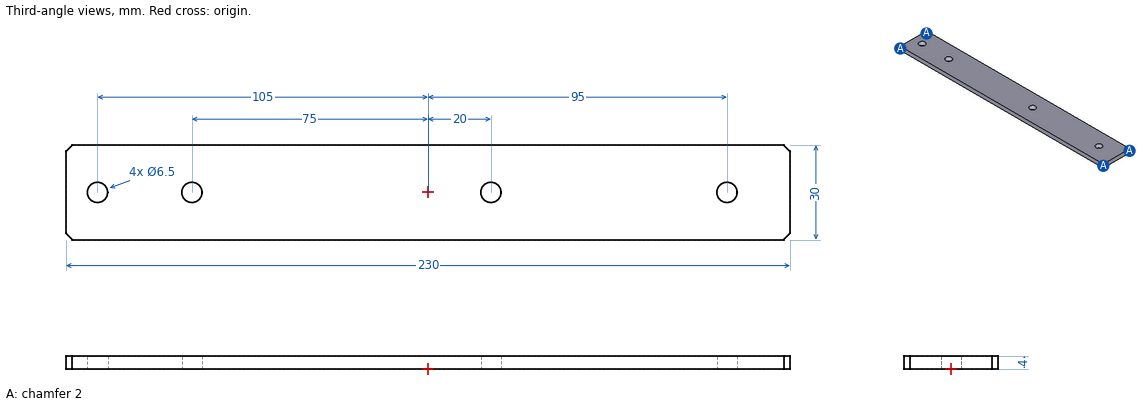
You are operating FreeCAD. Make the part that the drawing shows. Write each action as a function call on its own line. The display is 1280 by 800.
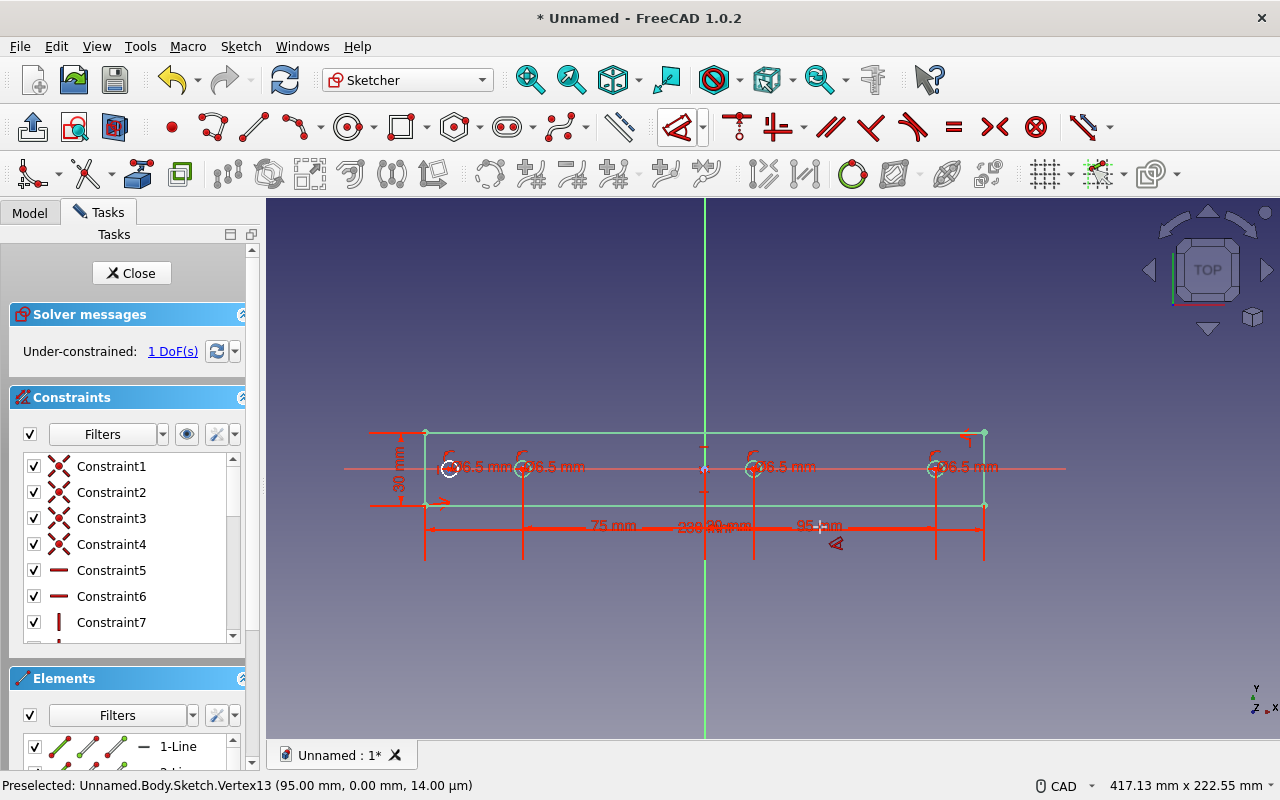
click(450, 469)
click(519, 527)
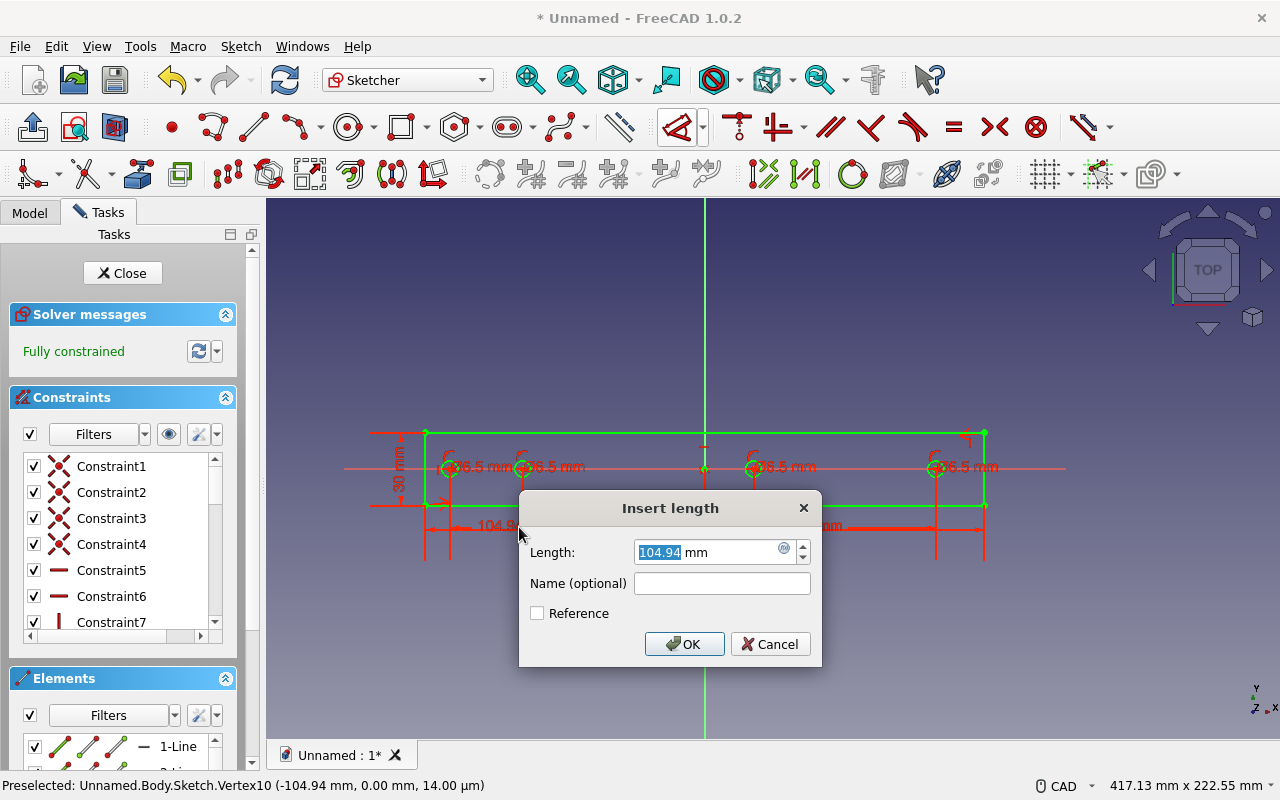
text(105)
key(Return)
key(Escape)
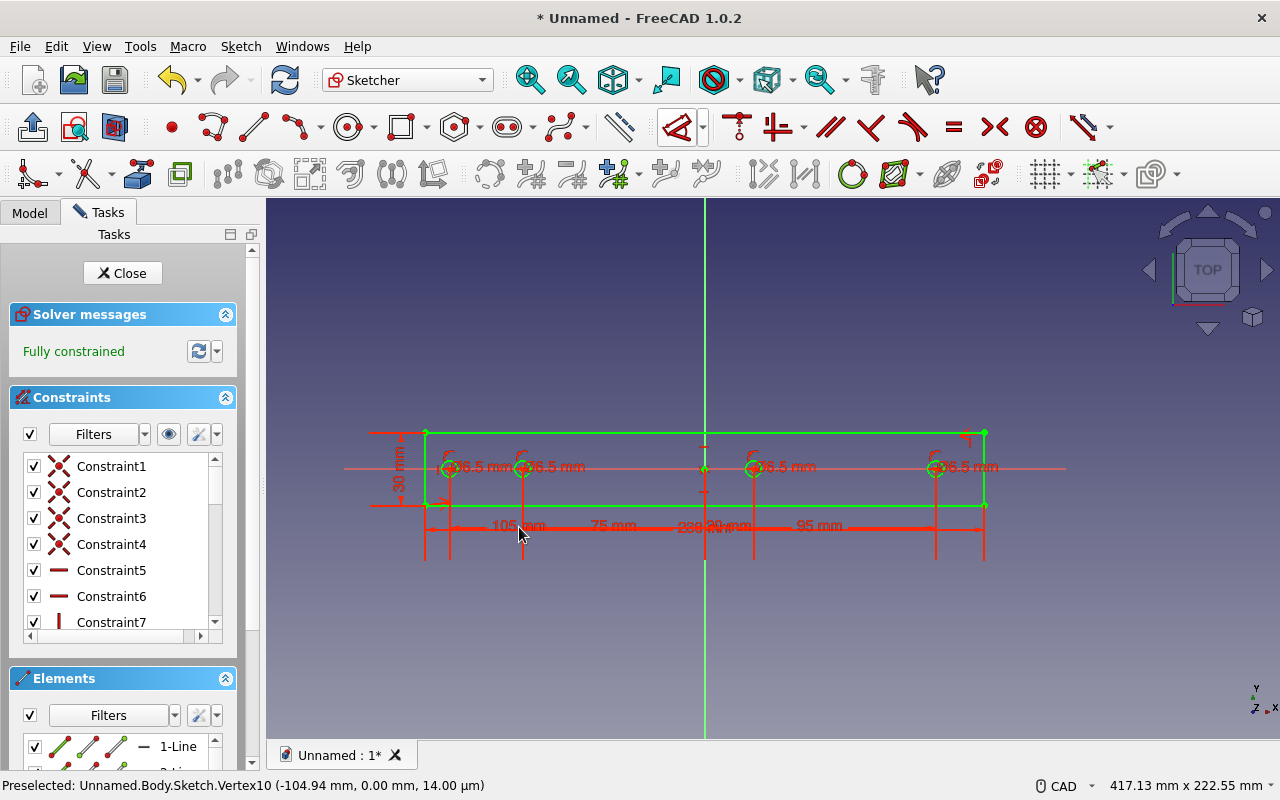
click(123, 273)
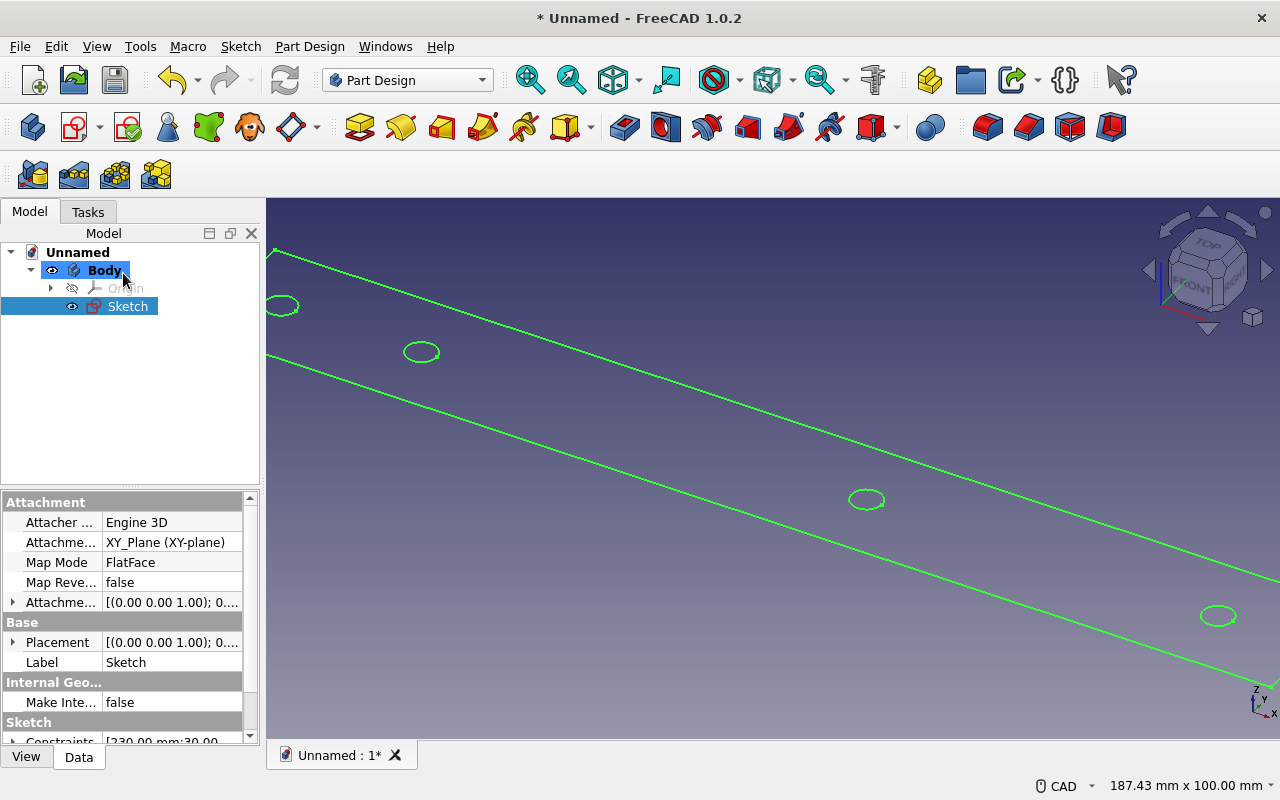
click(360, 128)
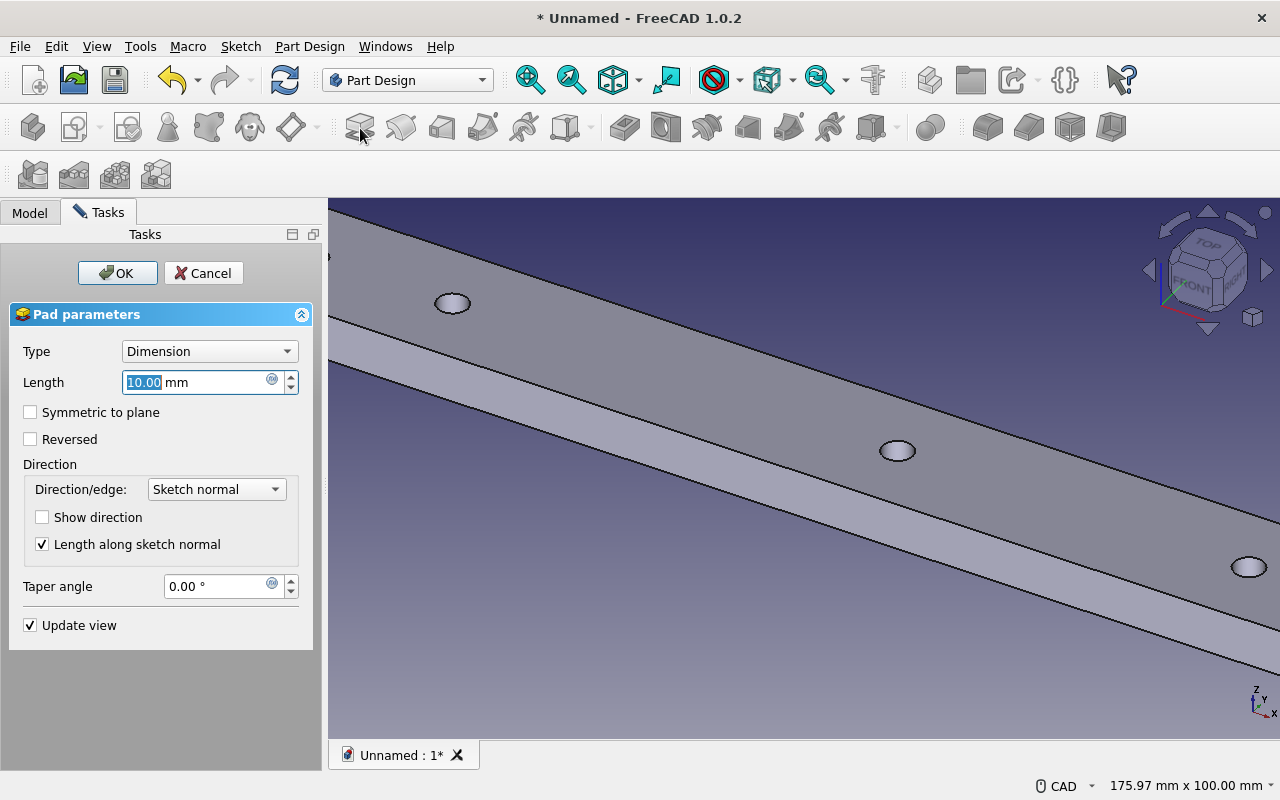
text(4)
key(Tab)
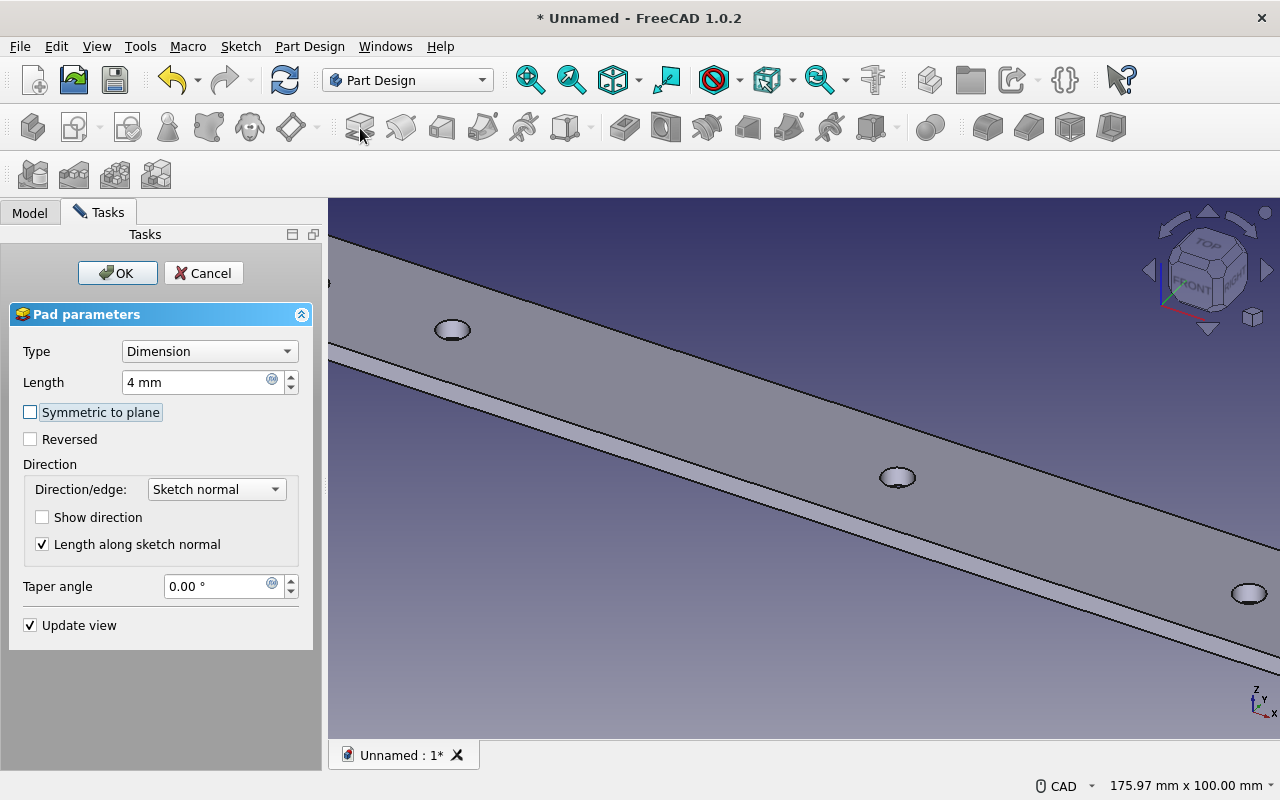
click(118, 273)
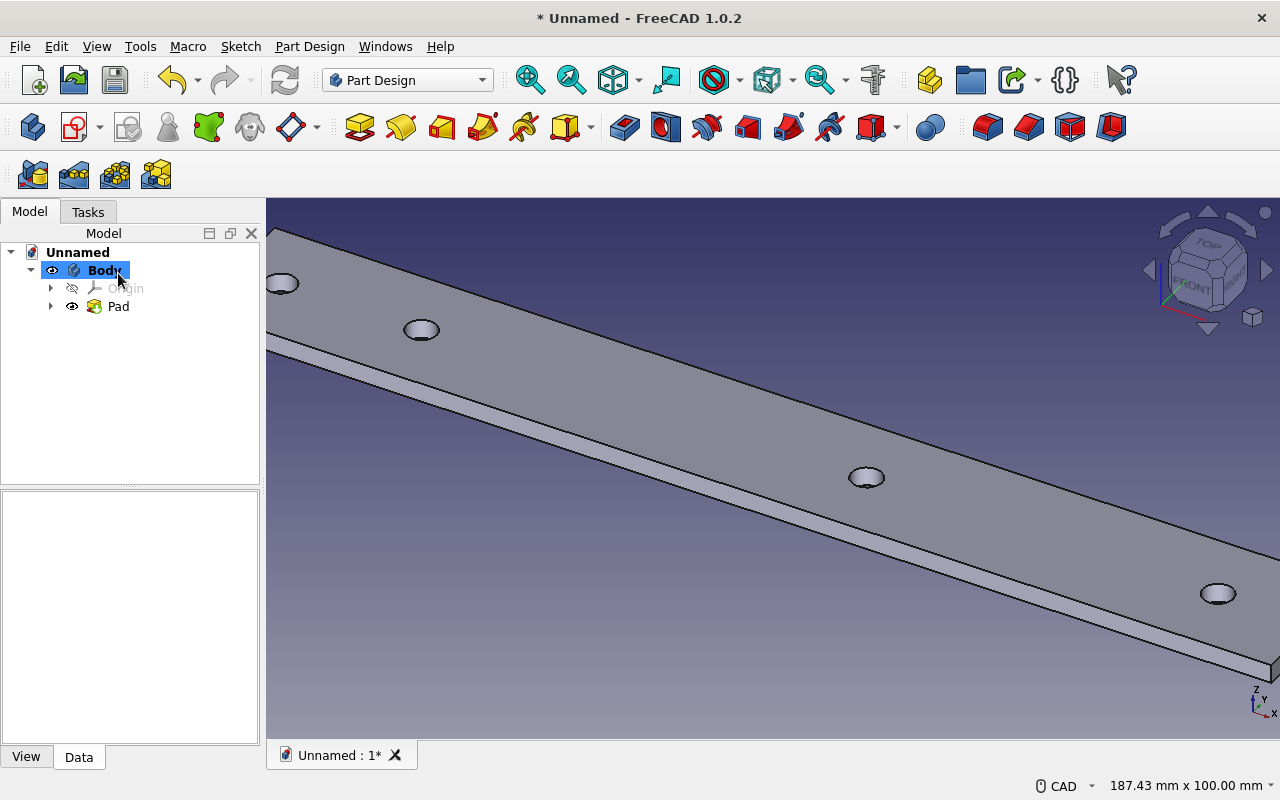
key(v)
key(f)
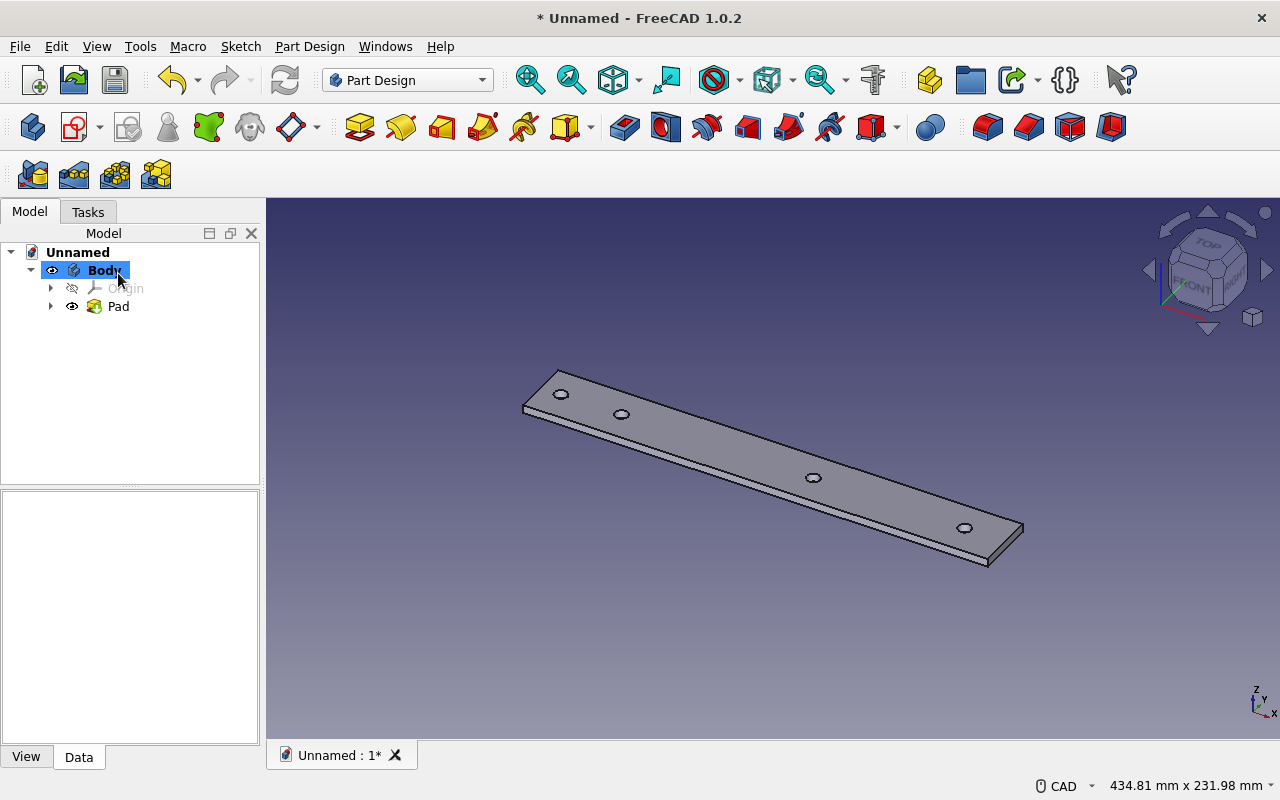
click(988, 564)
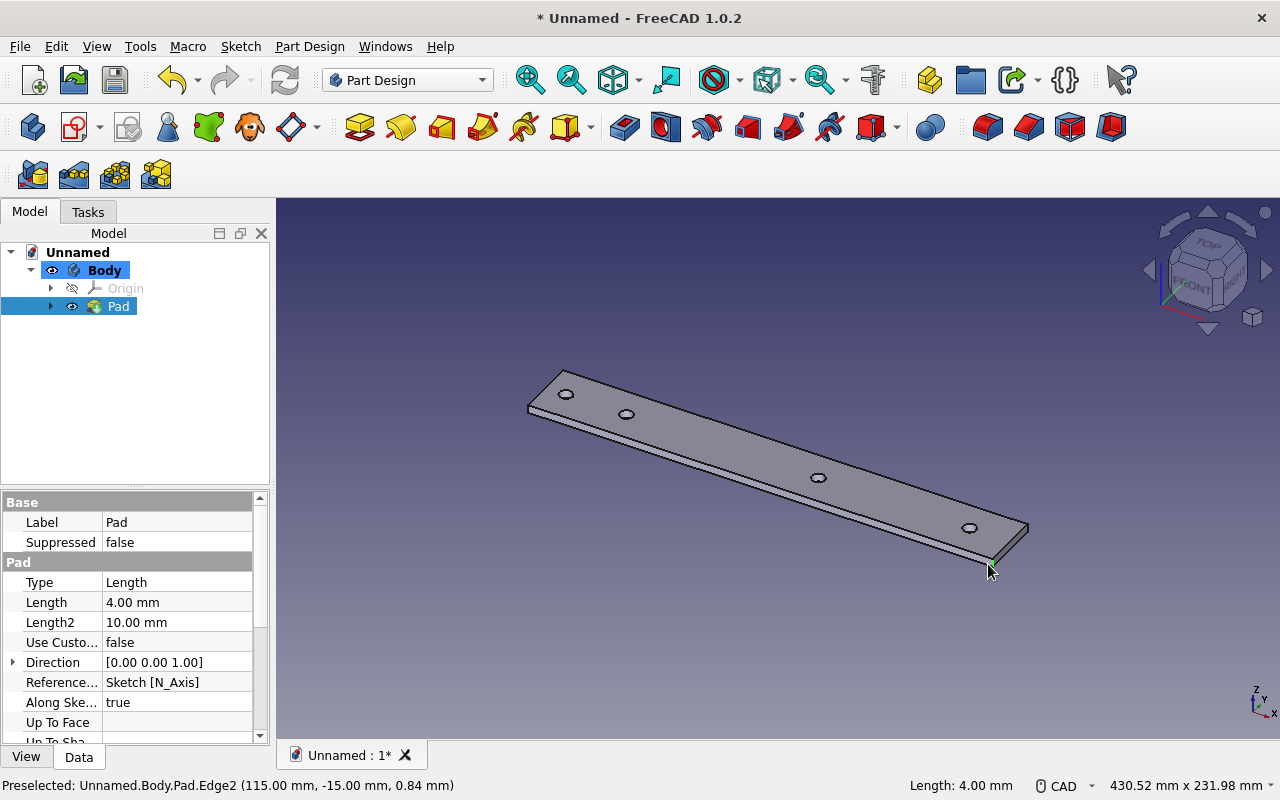
scroll(563, 373, up, 8)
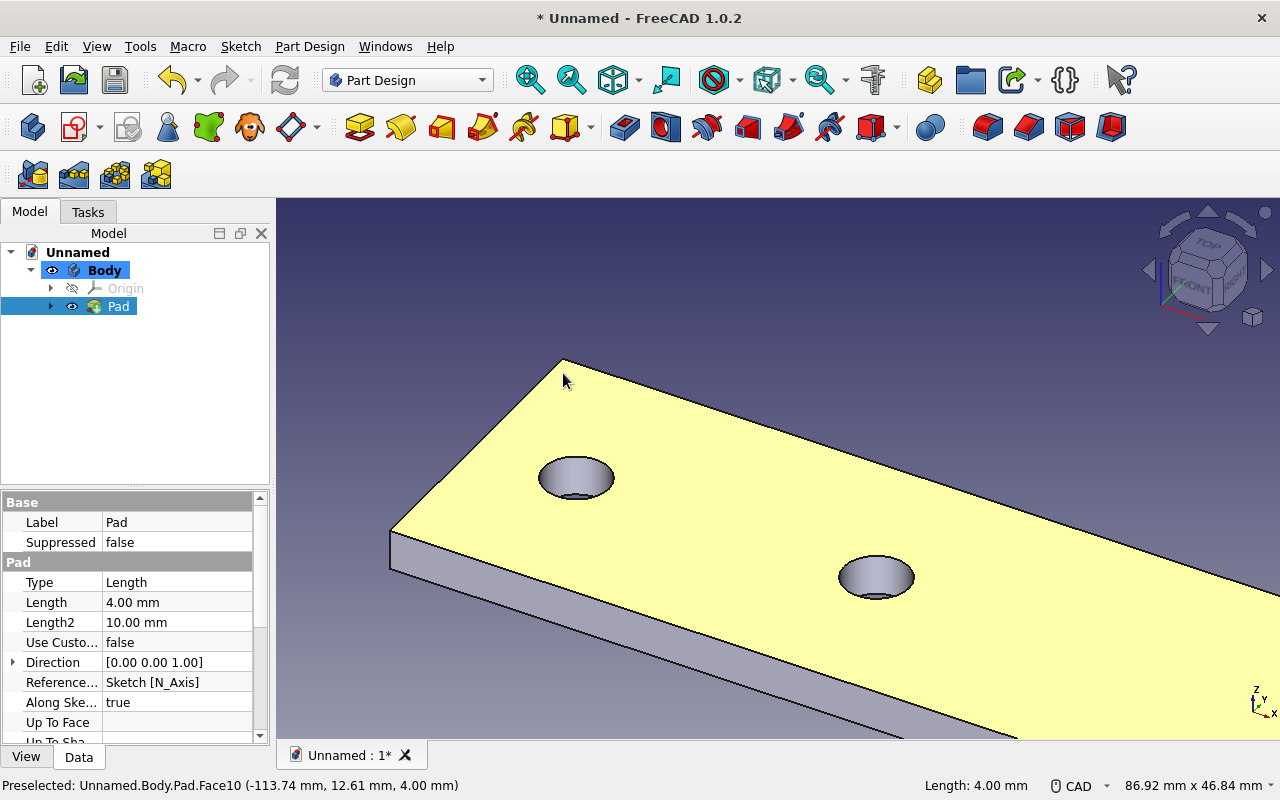
click(531, 80)